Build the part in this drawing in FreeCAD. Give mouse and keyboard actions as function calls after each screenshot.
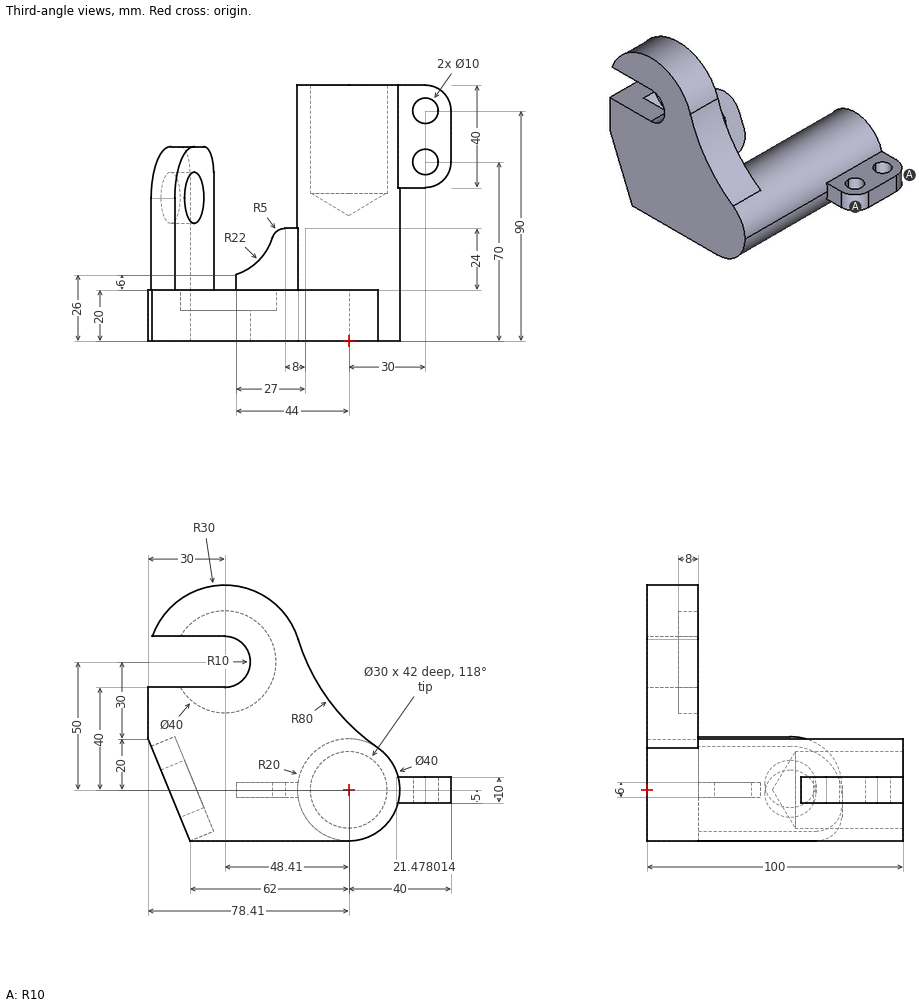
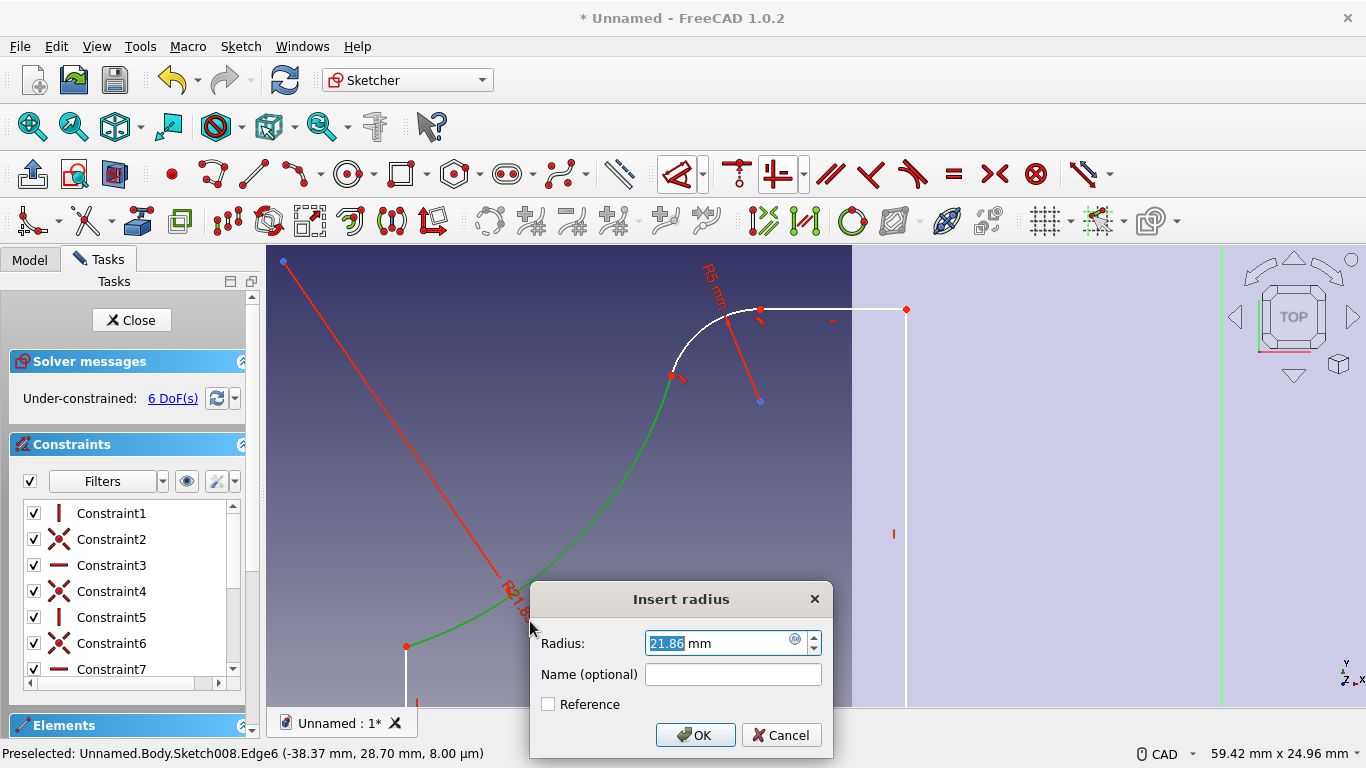
text(22)
key(Return)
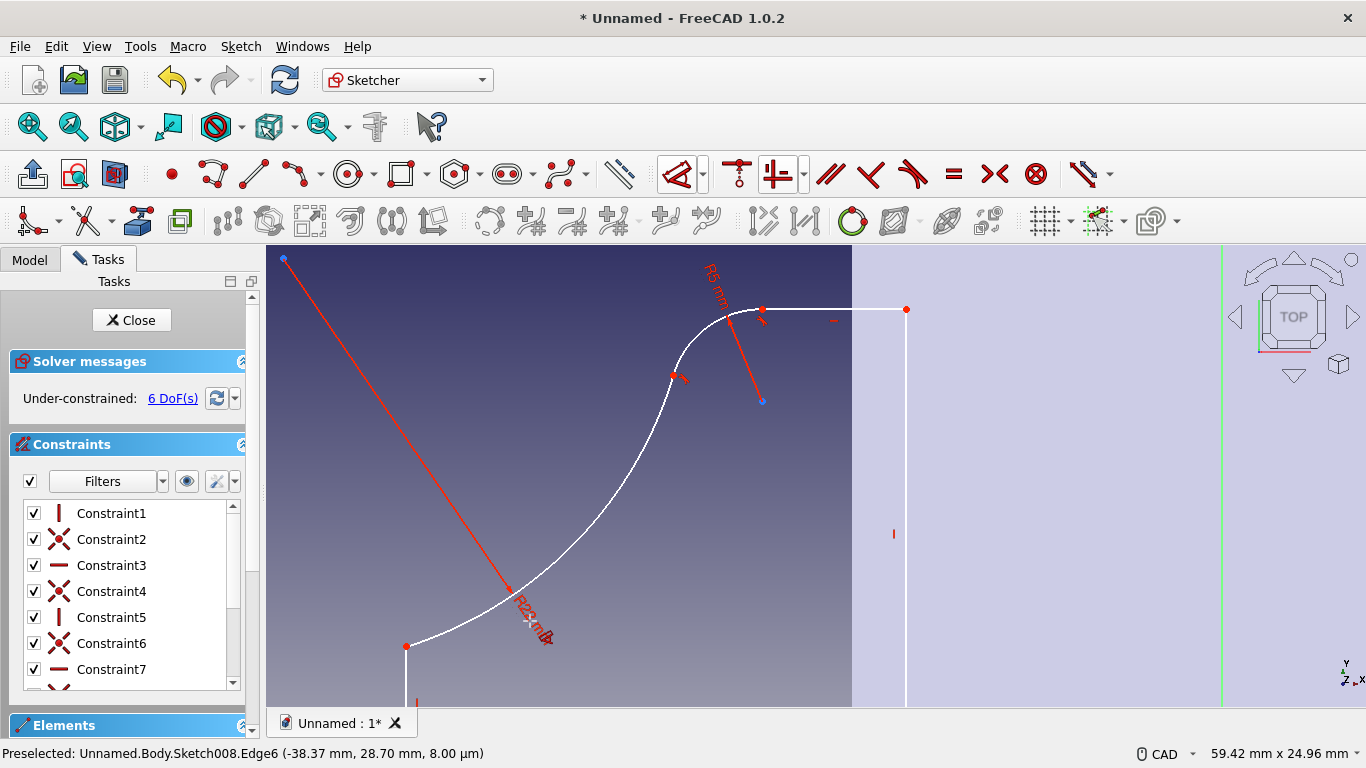
click(406, 669)
click(372, 663)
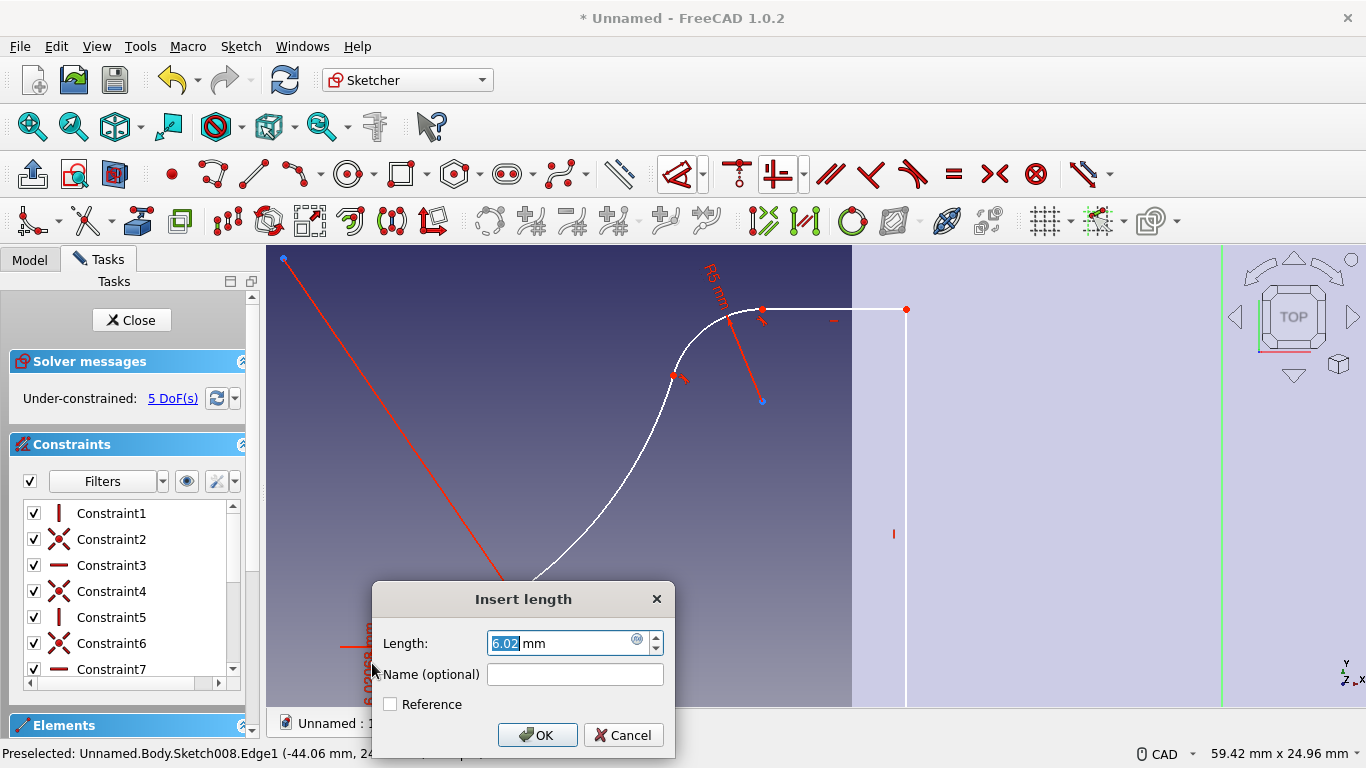
text(6)
key(Return)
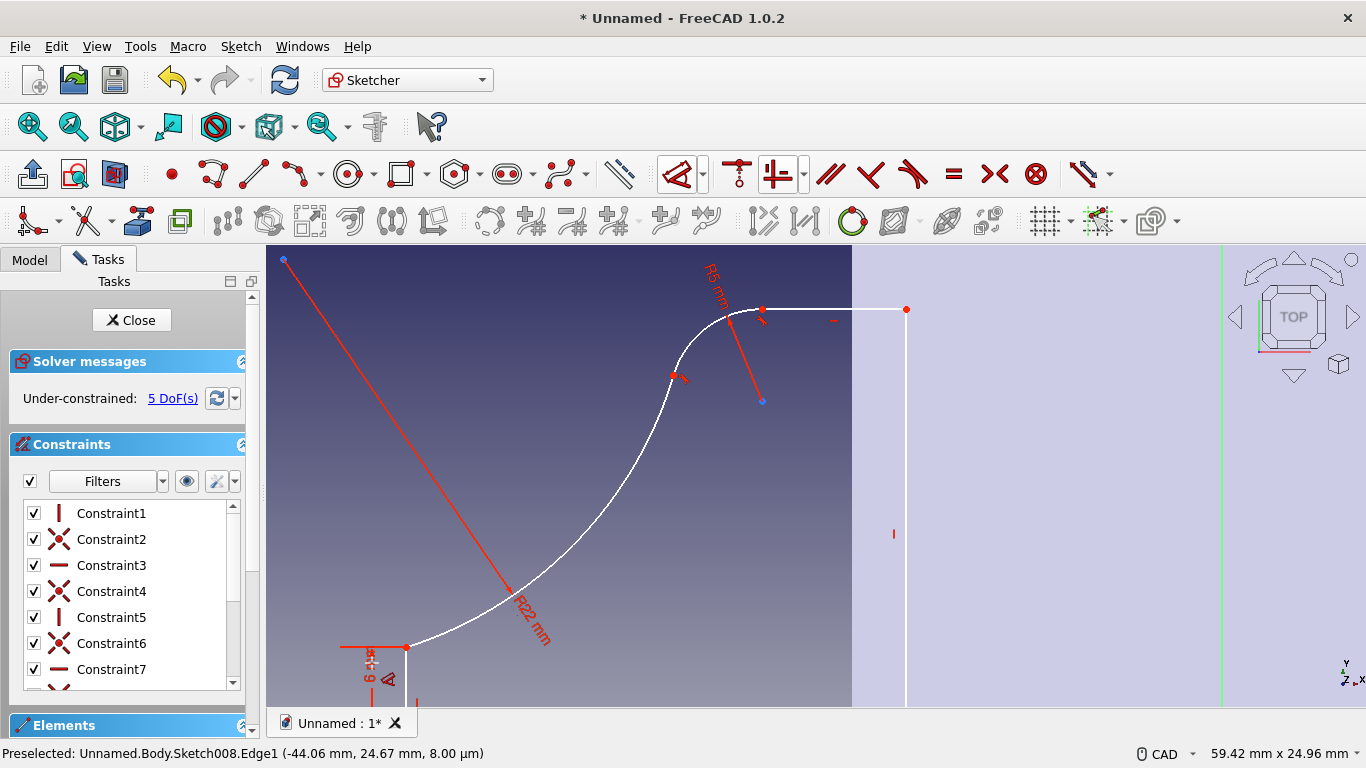
click(863, 309)
click(834, 275)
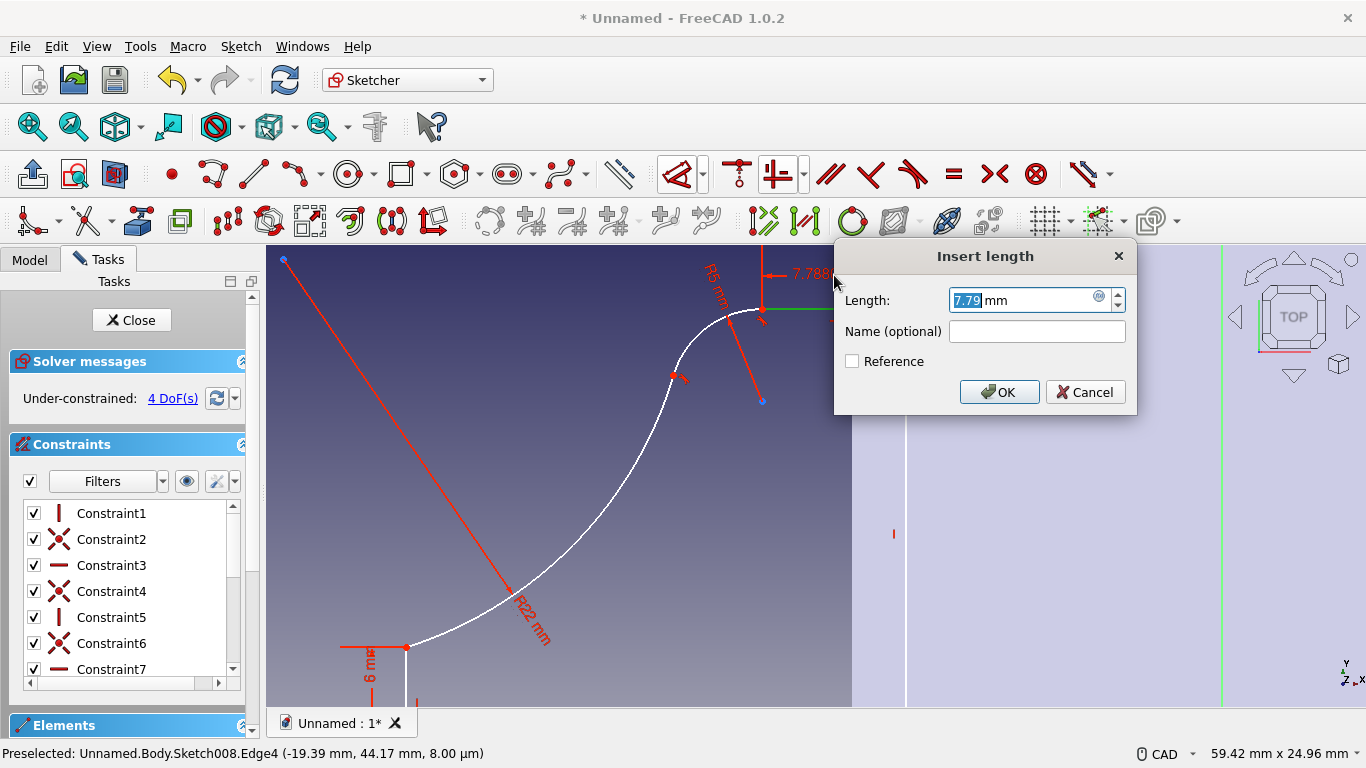
text(8)
key(Return)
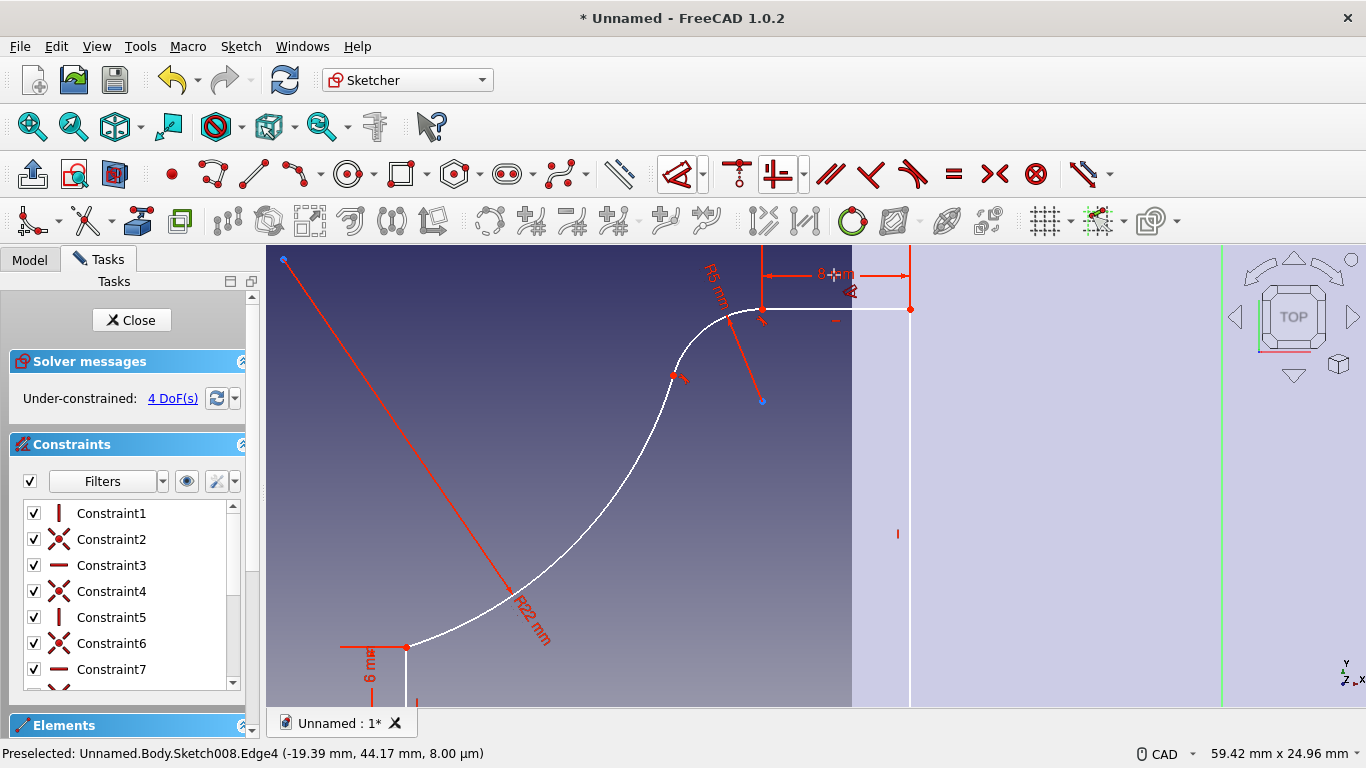
scroll(708, 334, down, 5)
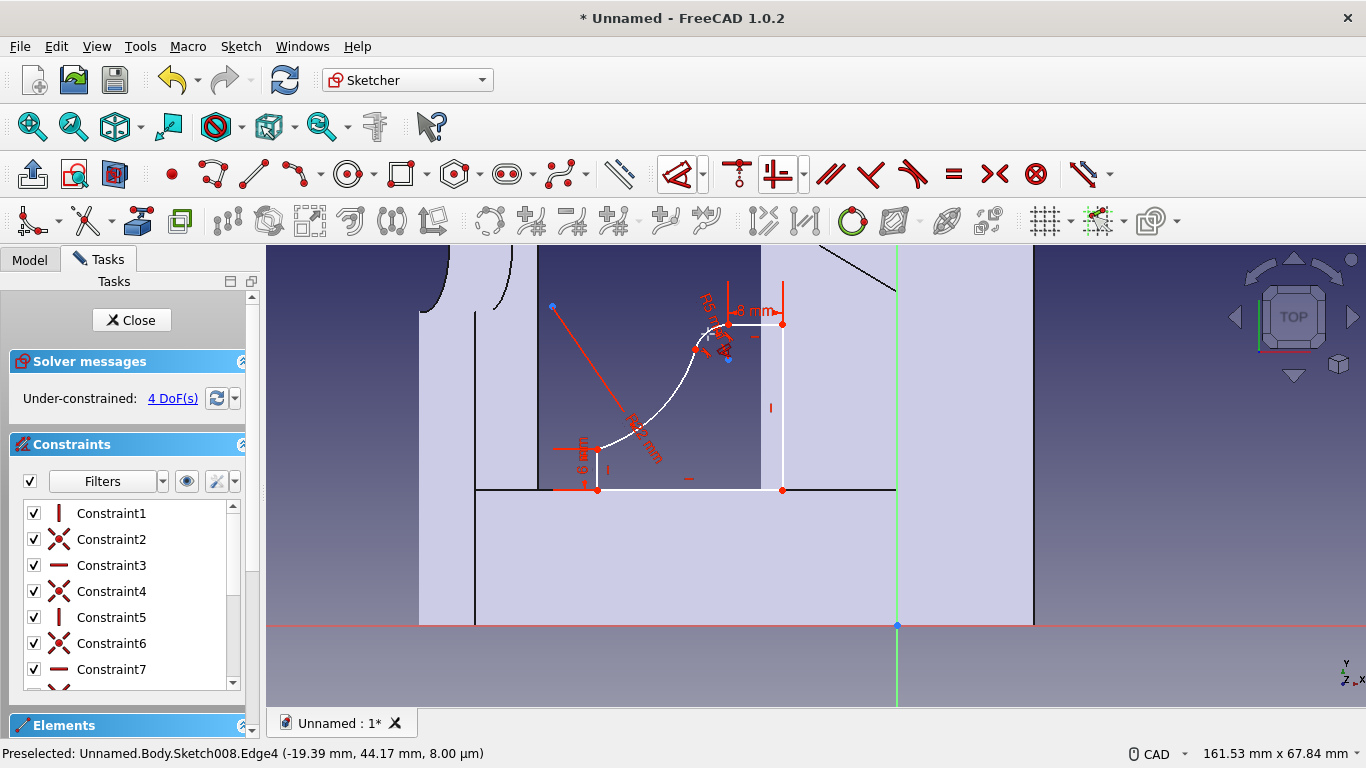
click(653, 490)
click(690, 524)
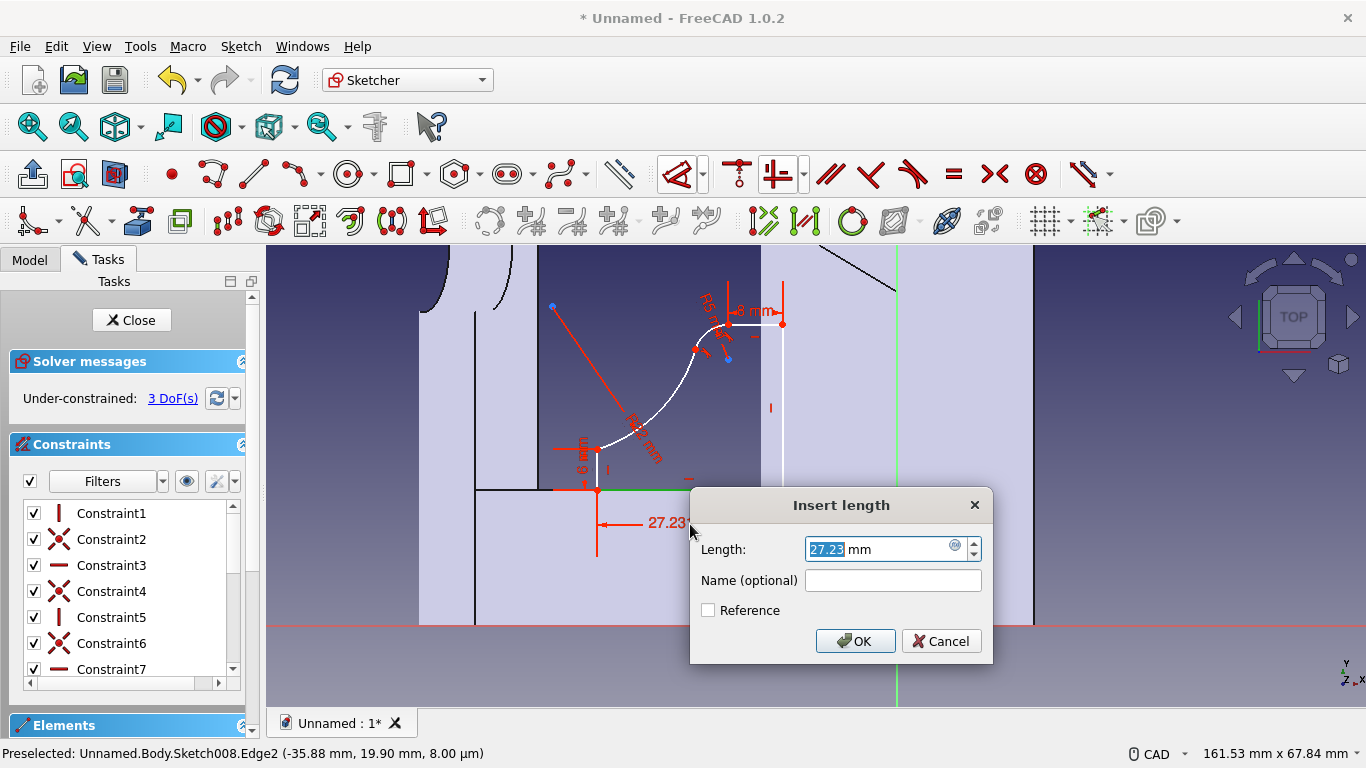
text(27)
key(Return)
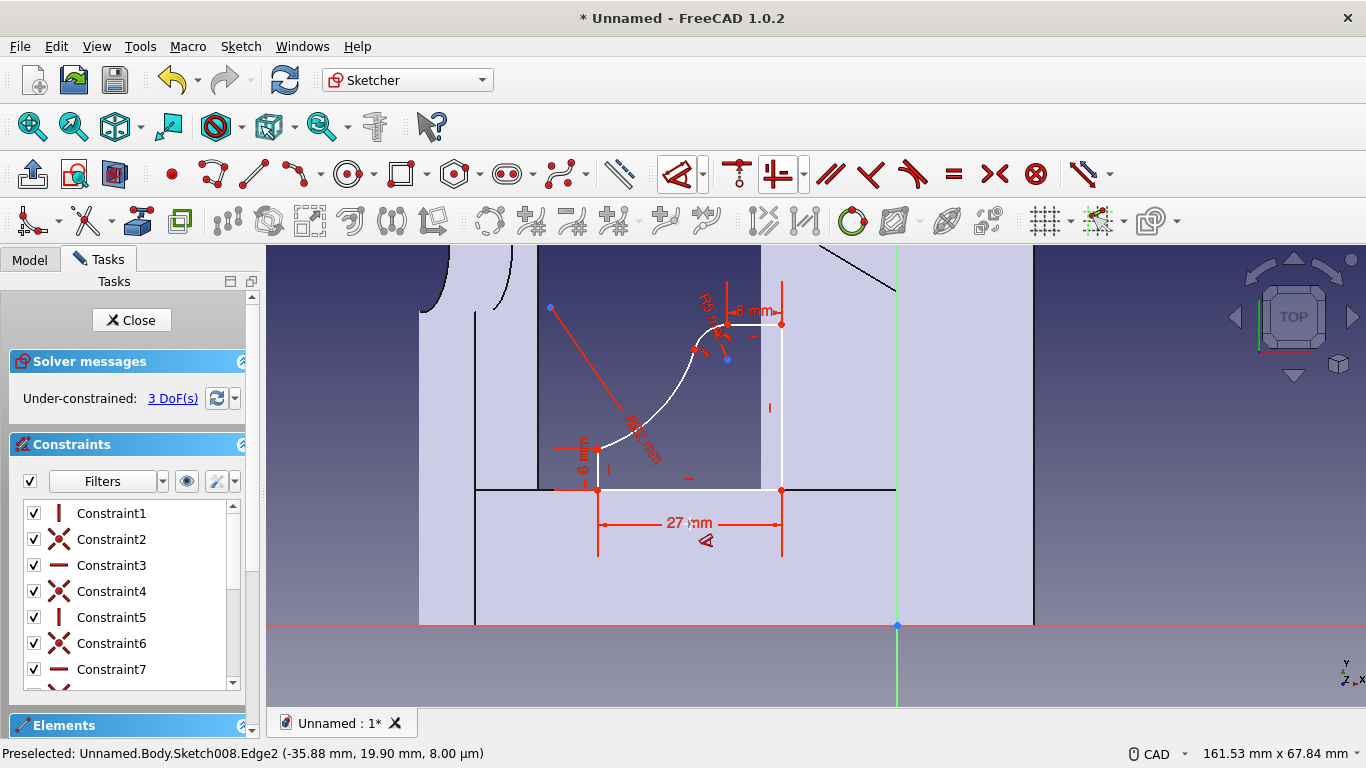
click(782, 441)
click(816, 408)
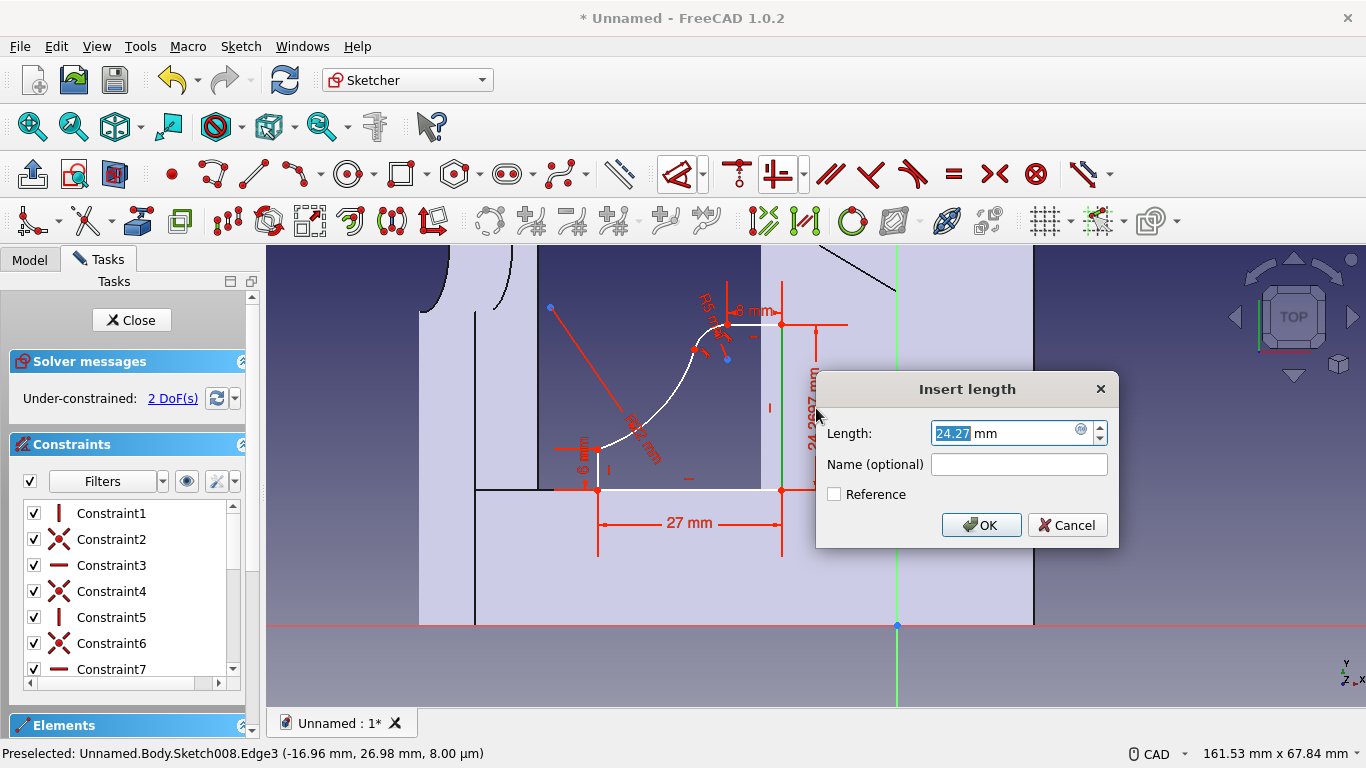
text(24)
key(Return)